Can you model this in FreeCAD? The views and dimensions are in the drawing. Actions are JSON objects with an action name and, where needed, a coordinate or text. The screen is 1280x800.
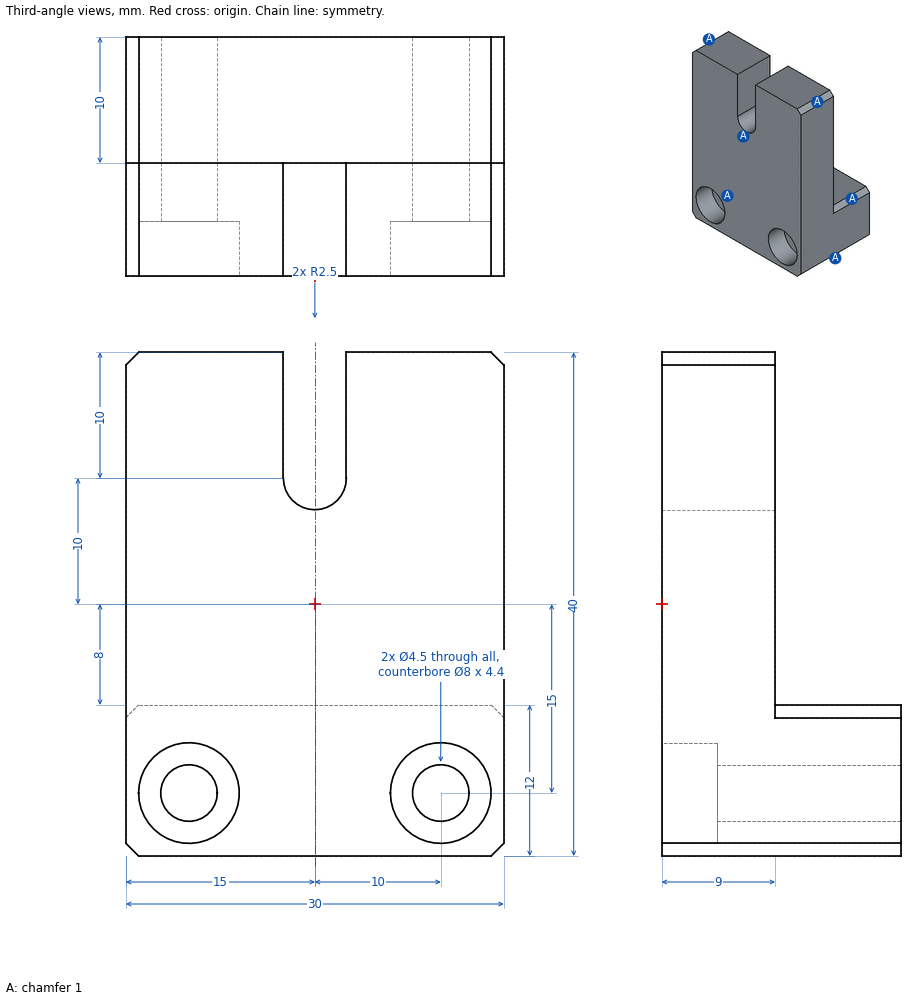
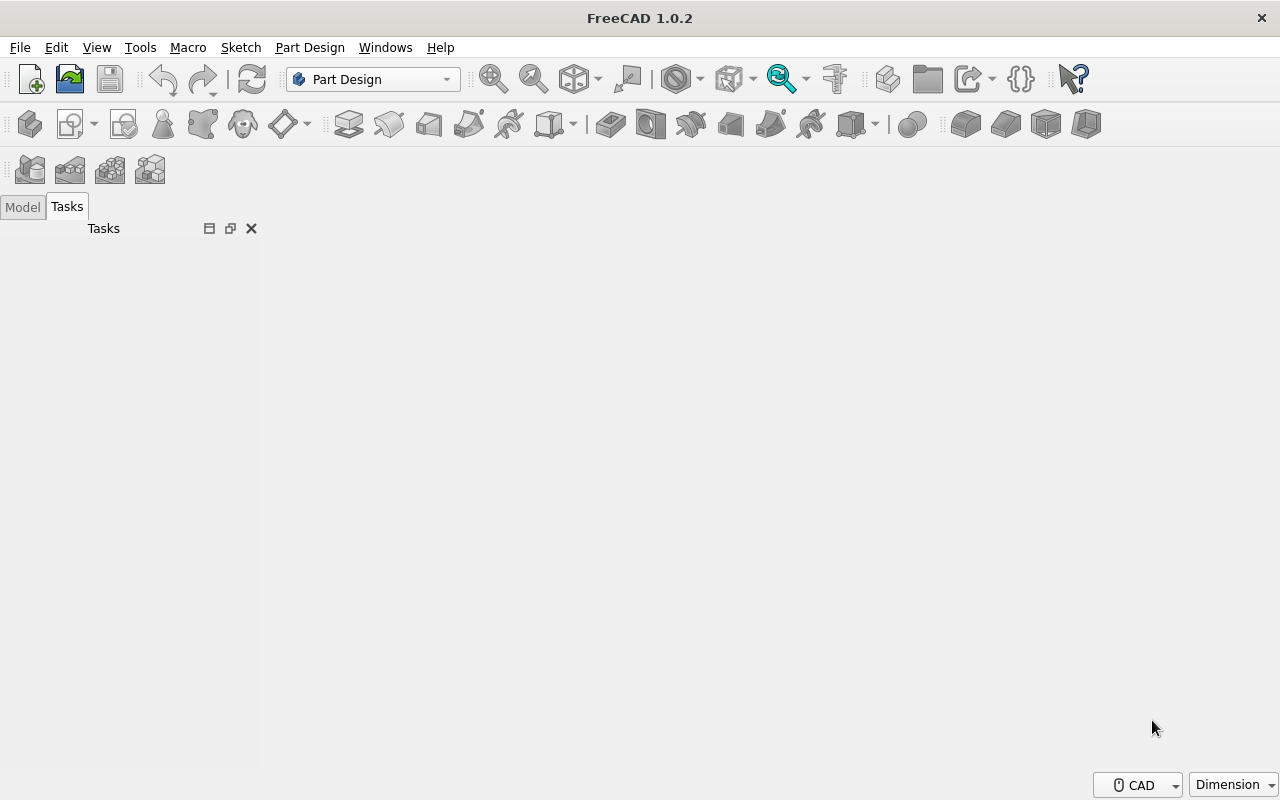
{"action": "key", "text": "ctrl+n"}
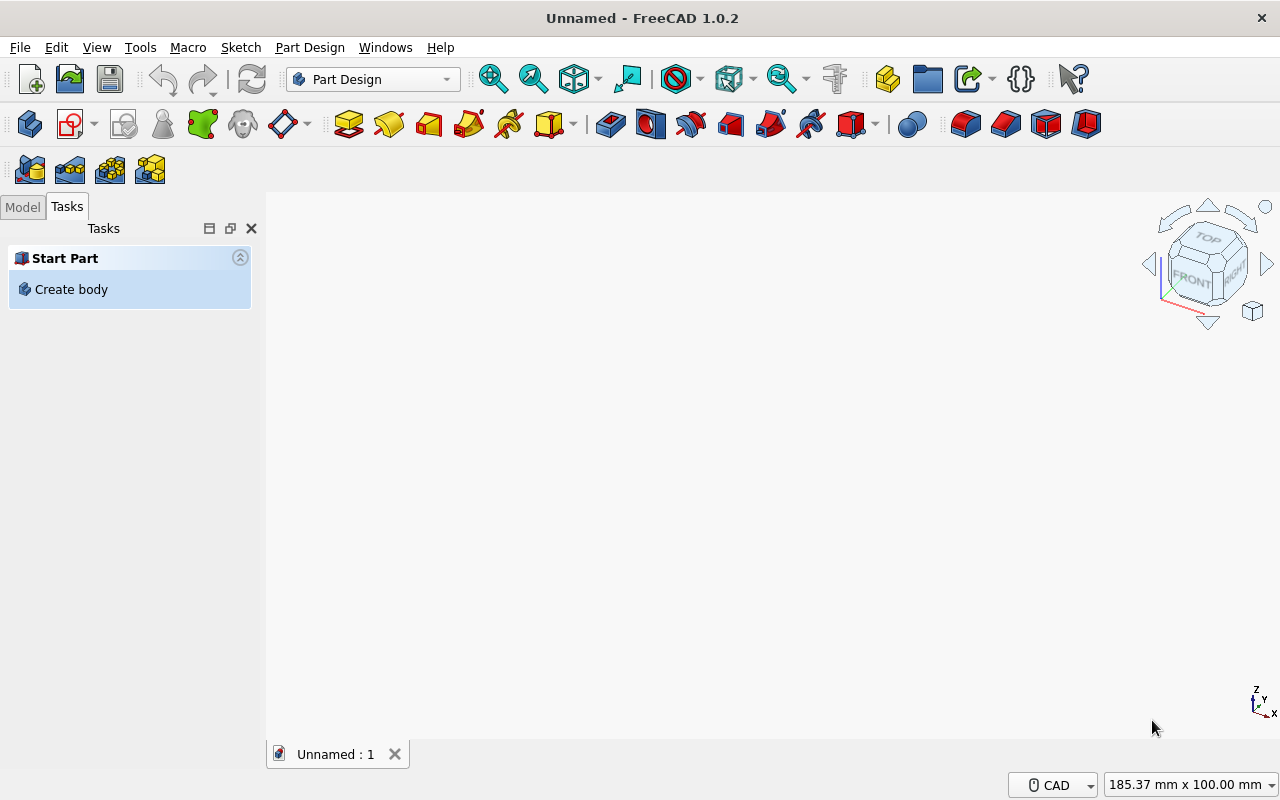
{"action": "left_click", "coordinate": [70, 124]}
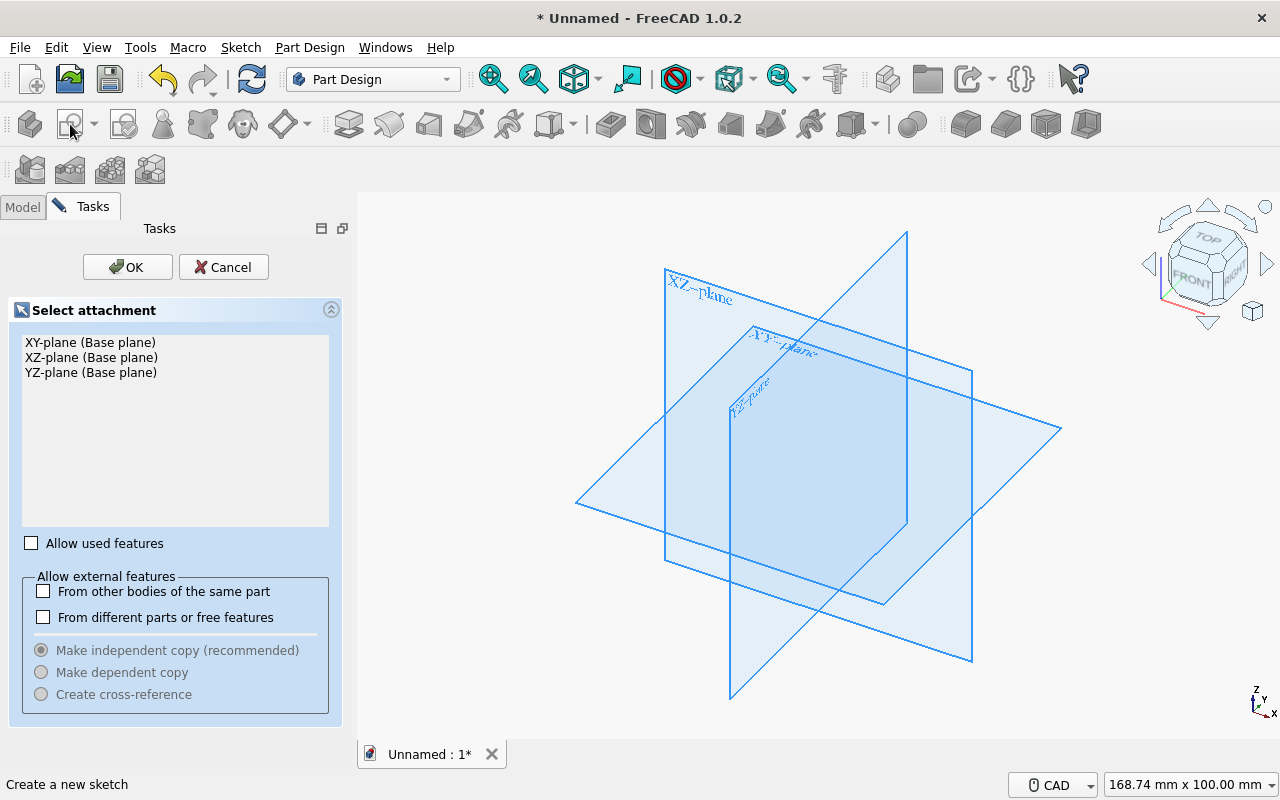
{"action": "left_click", "coordinate": [82, 358]}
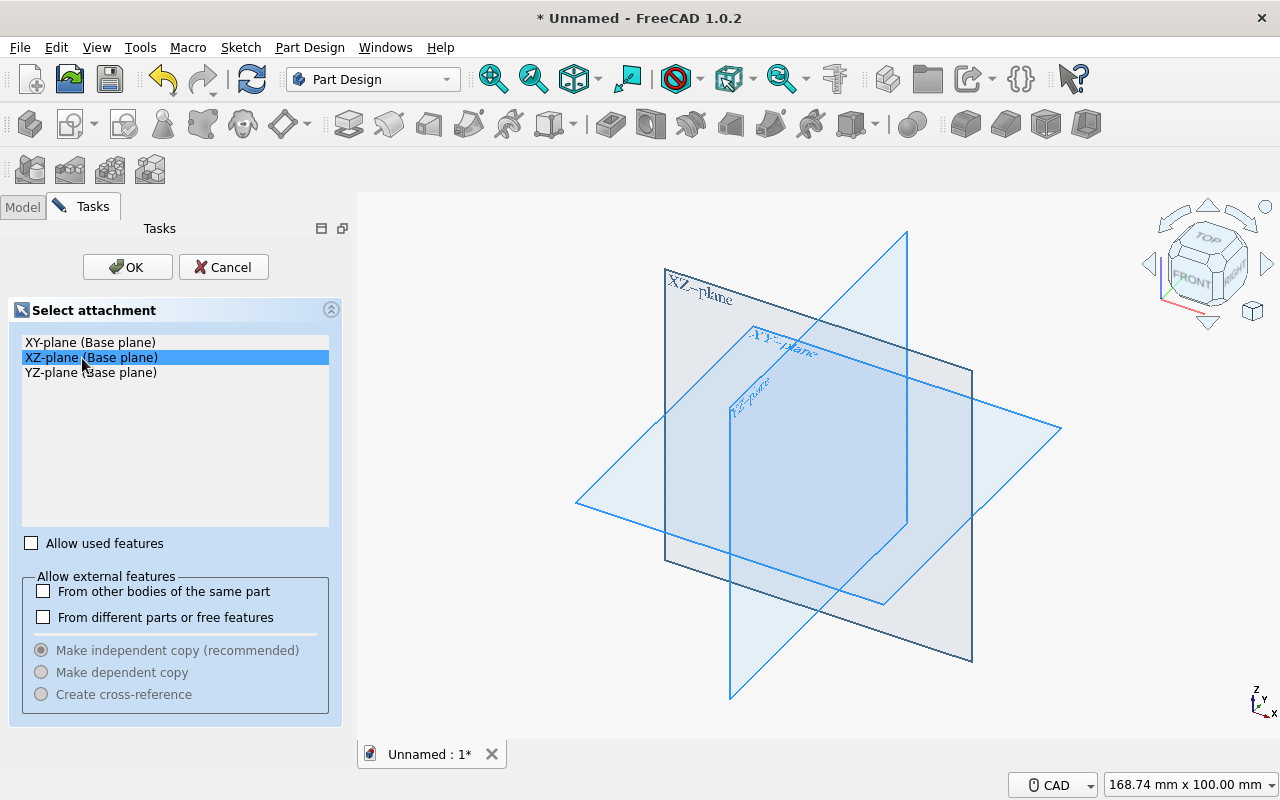
{"action": "left_click", "coordinate": [128, 267]}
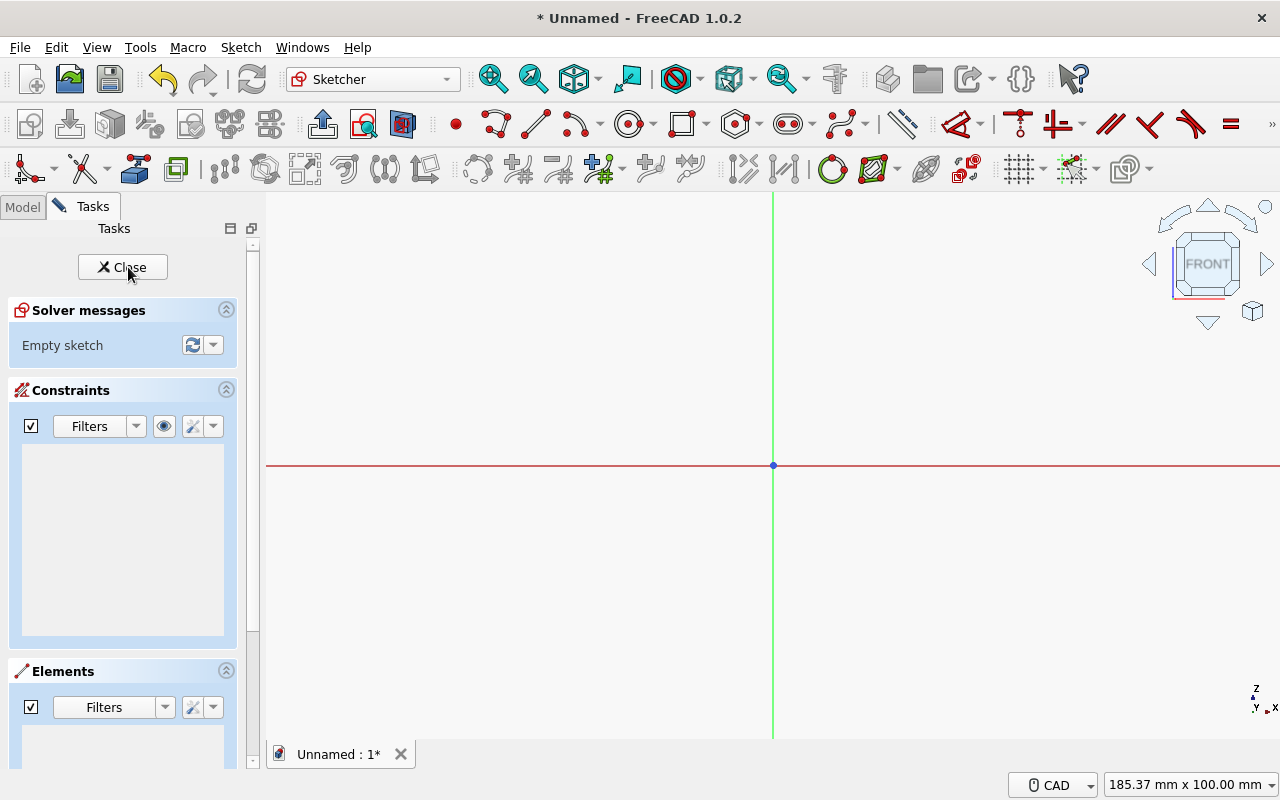
{"action": "scroll", "coordinate": [912, 466], "scroll_direction": "up", "scroll_amount": 2}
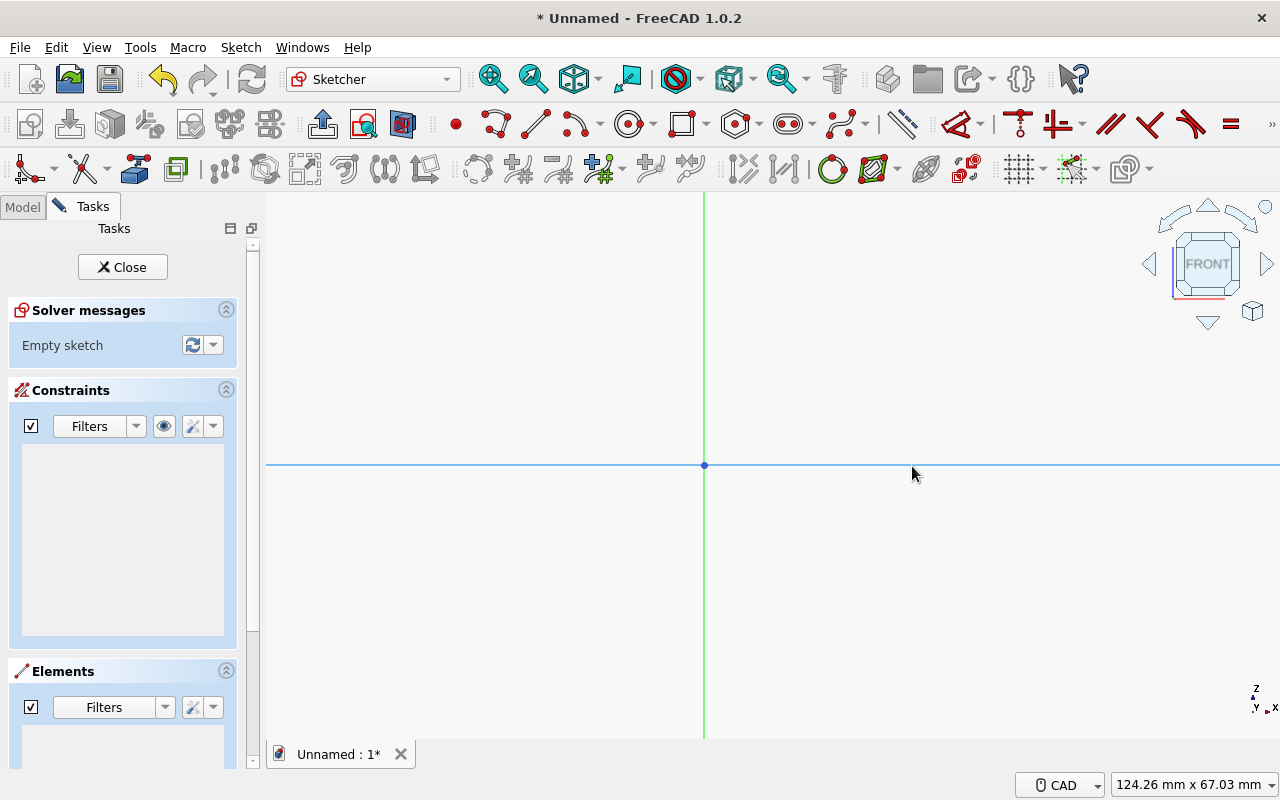
{"action": "key", "text": "g v"}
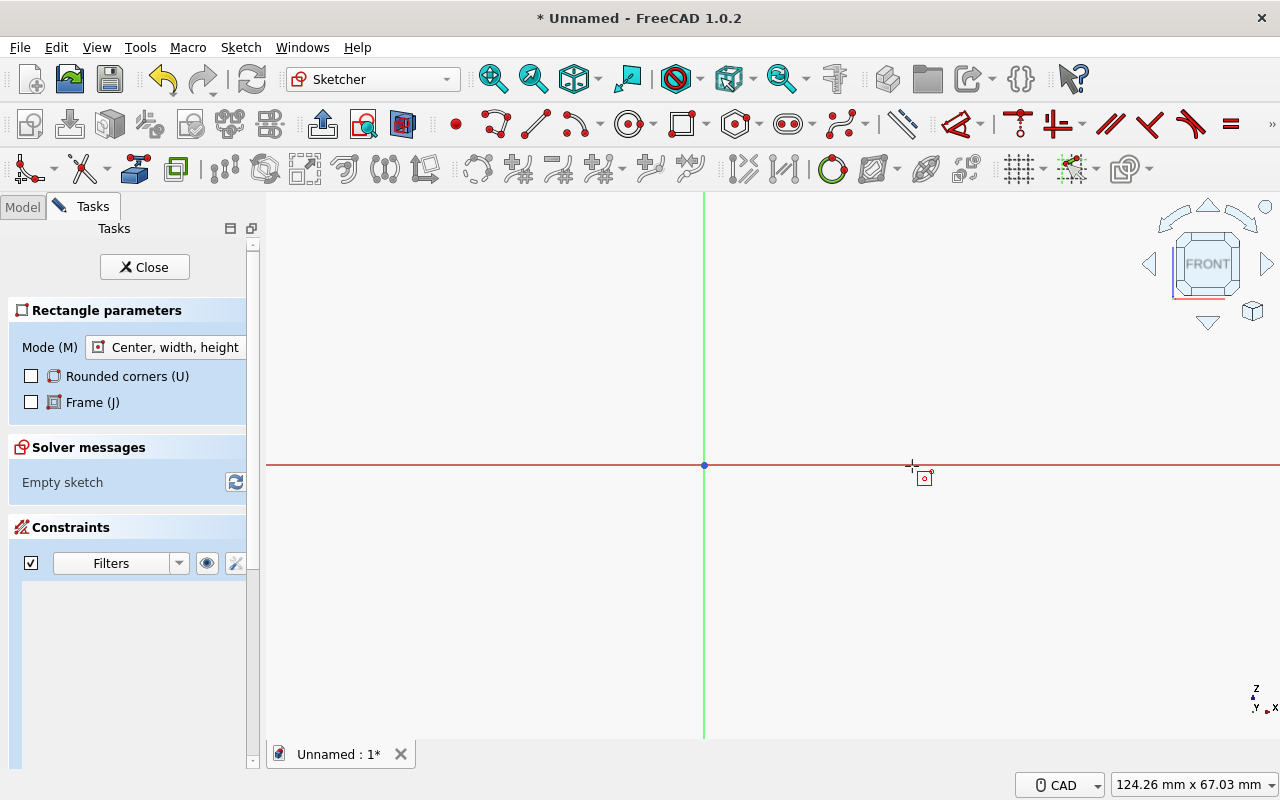
{"action": "left_click", "coordinate": [704, 465]}
{"action": "mouse_move", "coordinate": [827, 302]}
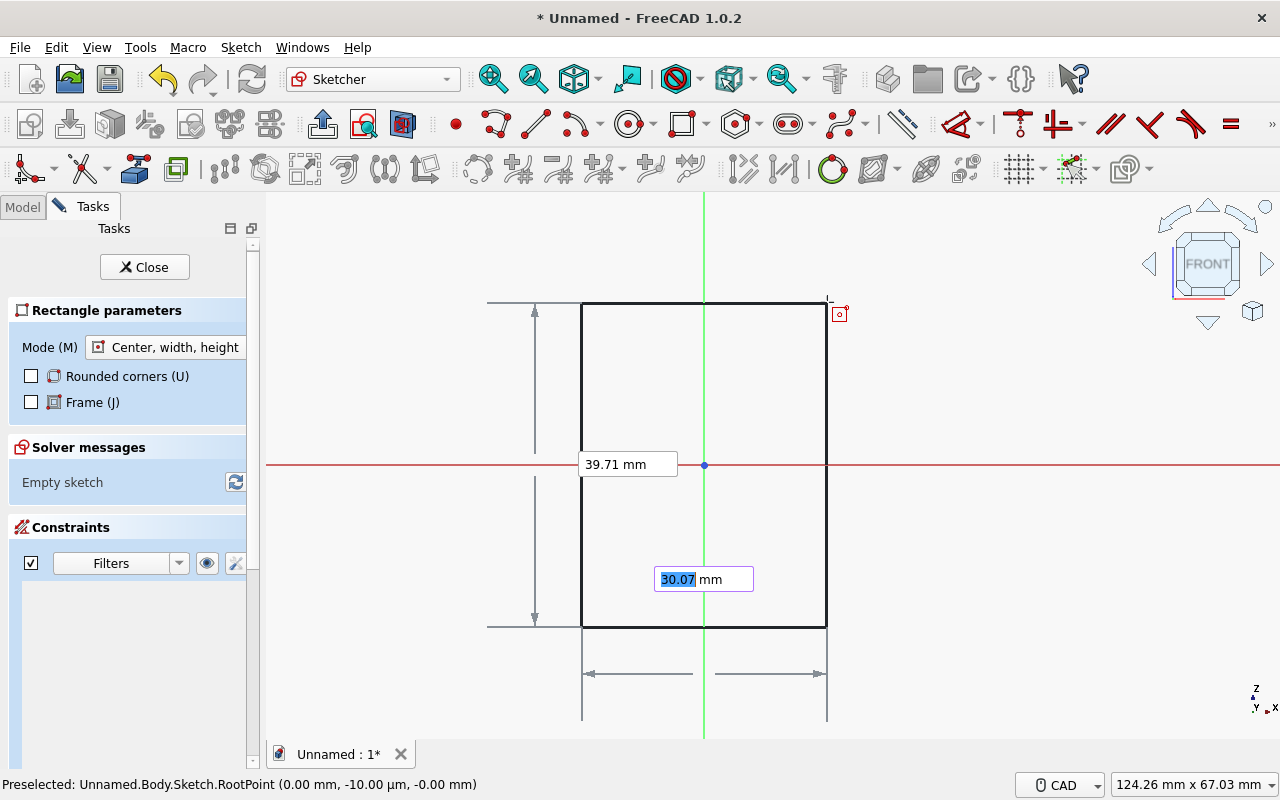
{"action": "type", "text": "30"}
{"action": "key", "text": "Tab"}
{"action": "type", "text": "40"}
{"action": "key", "text": "Return"}
{"action": "key", "text": "Escape"}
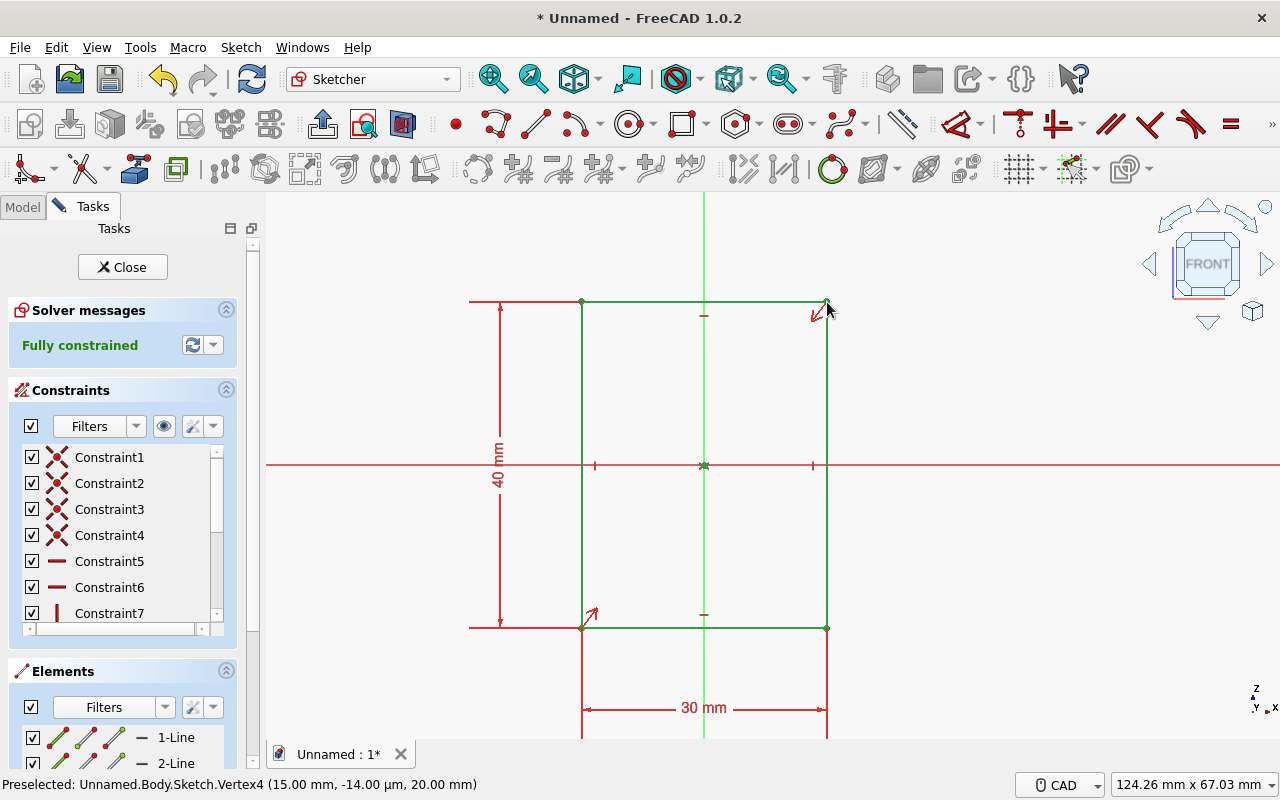
{"action": "left_click", "coordinate": [123, 267]}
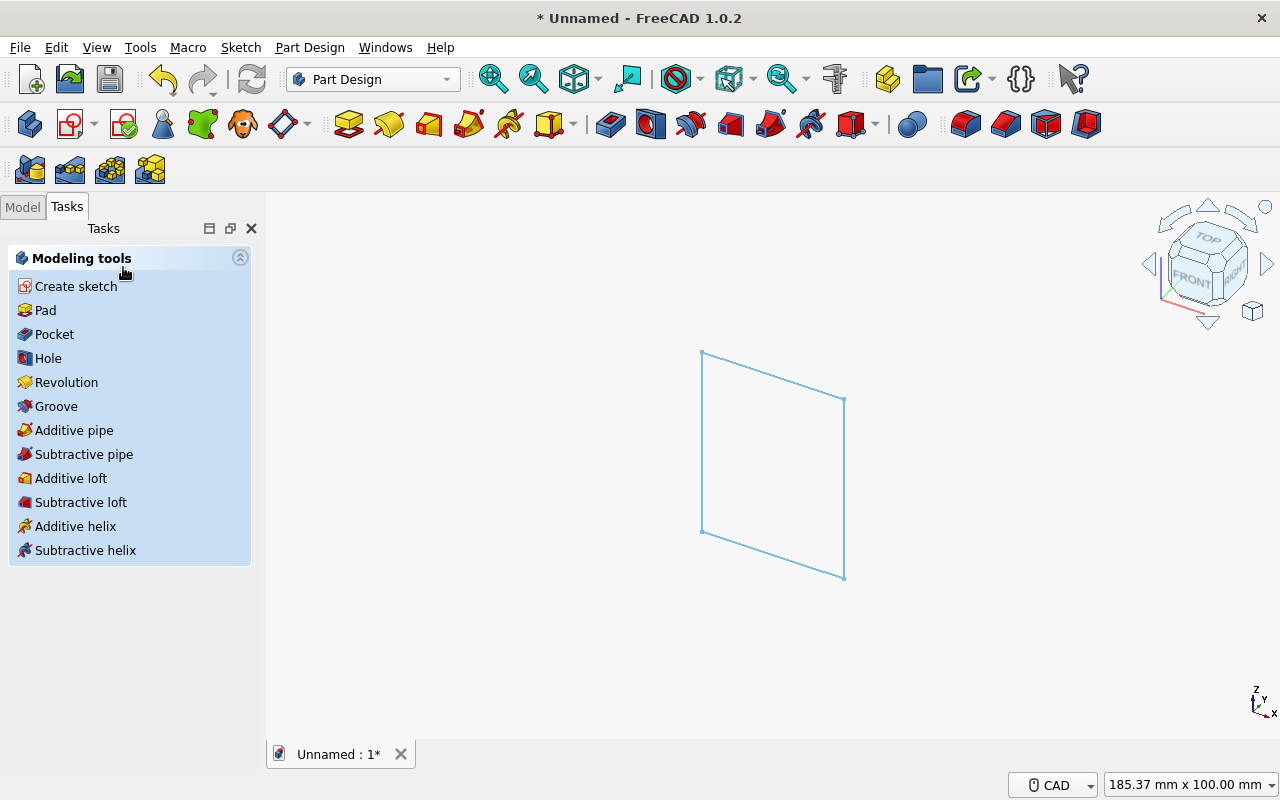
{"action": "left_click", "coordinate": [350, 124]}